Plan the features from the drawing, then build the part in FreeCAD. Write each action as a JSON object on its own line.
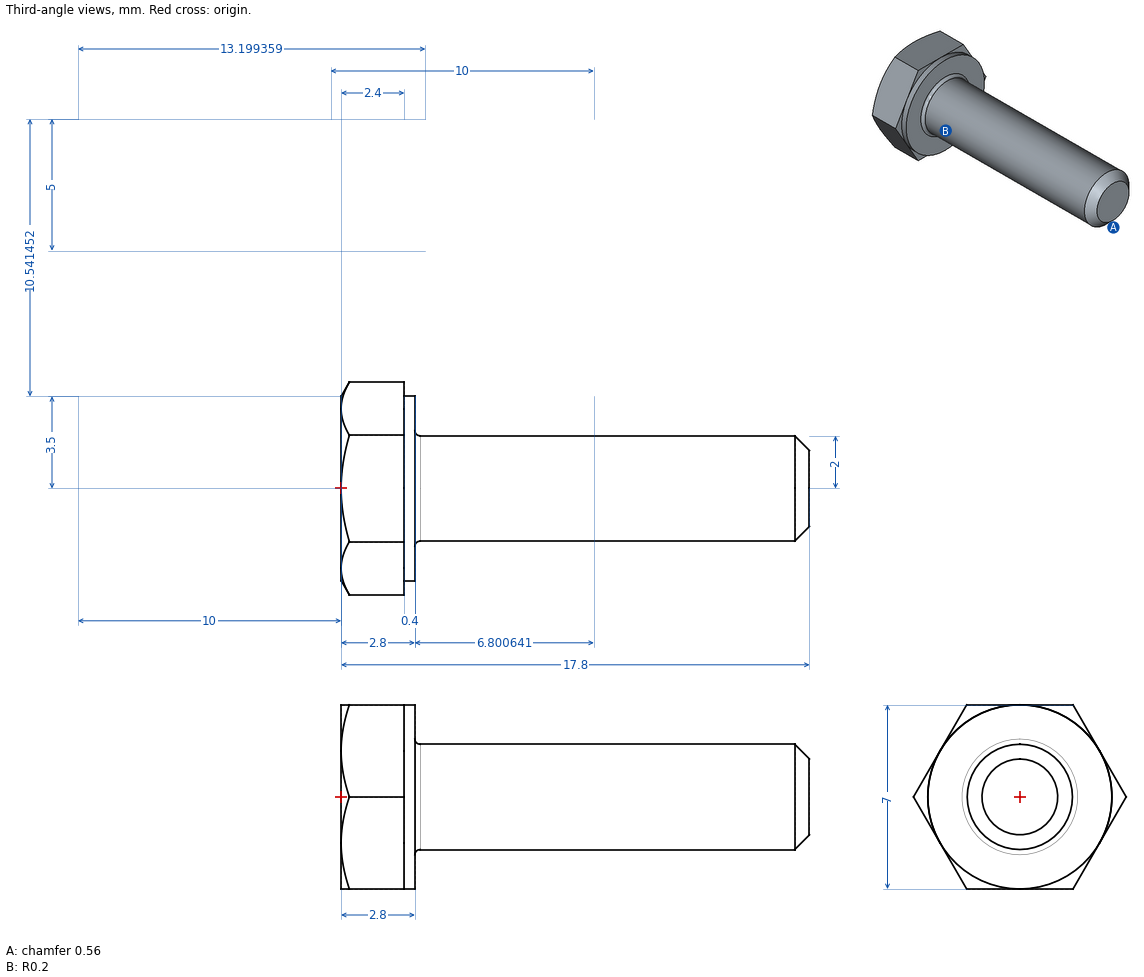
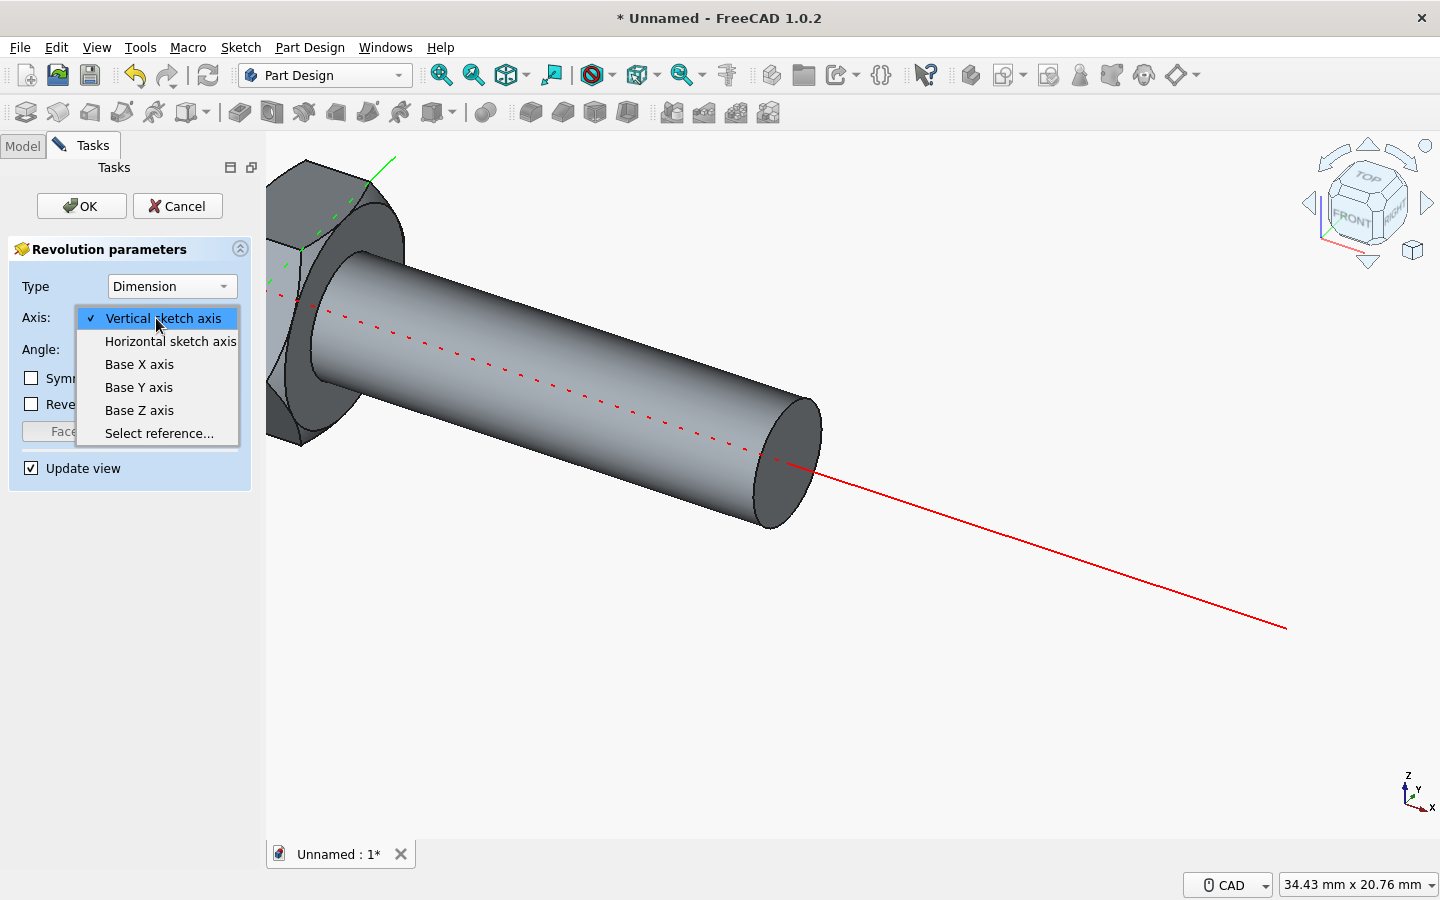
{"action": "left_click", "coordinate": [156, 342]}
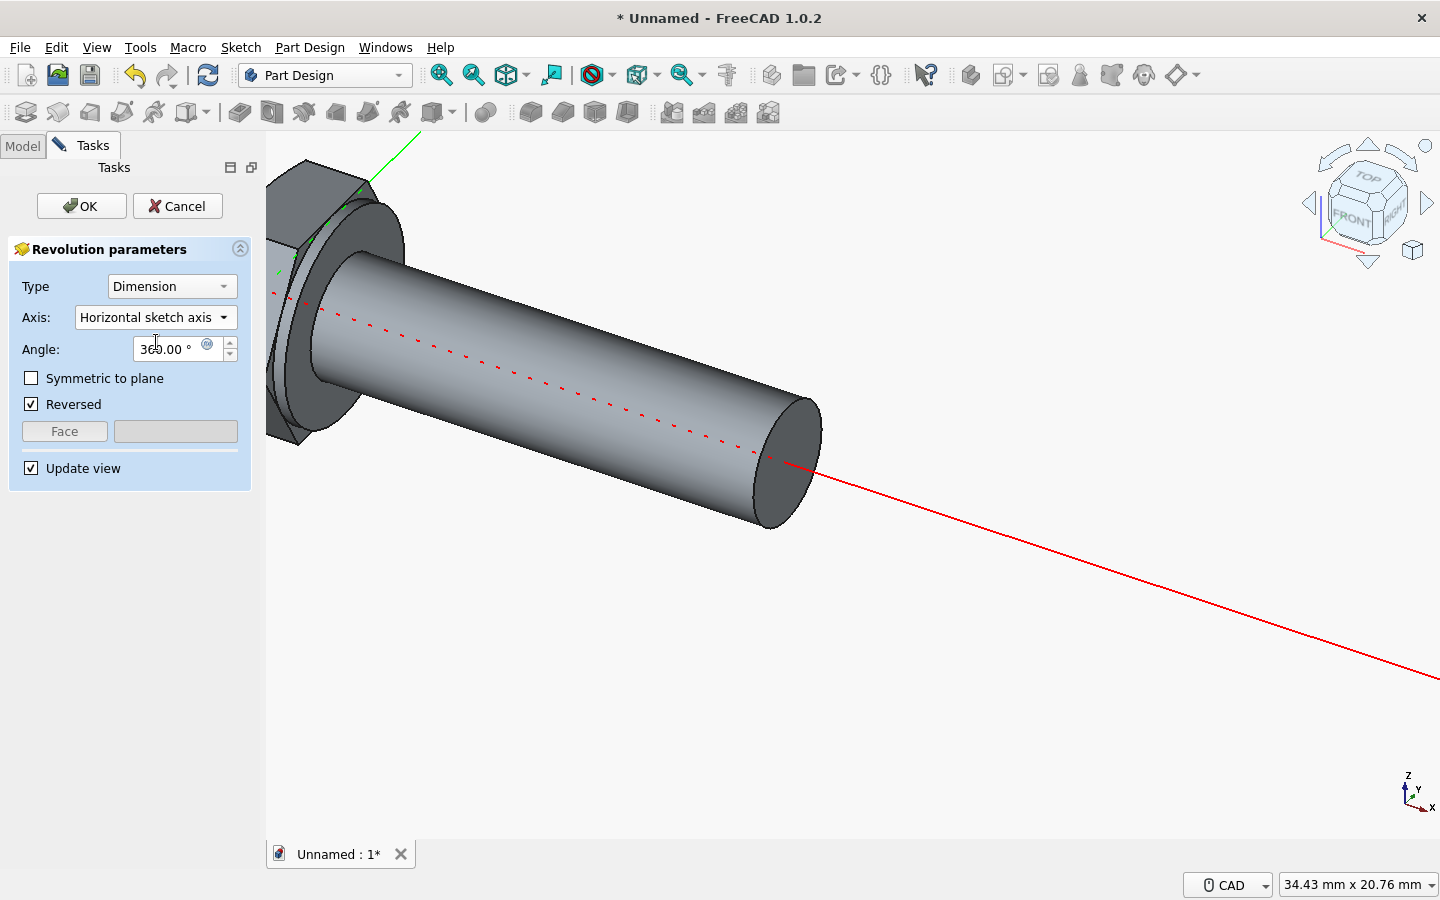
{"action": "left_click", "coordinate": [82, 206]}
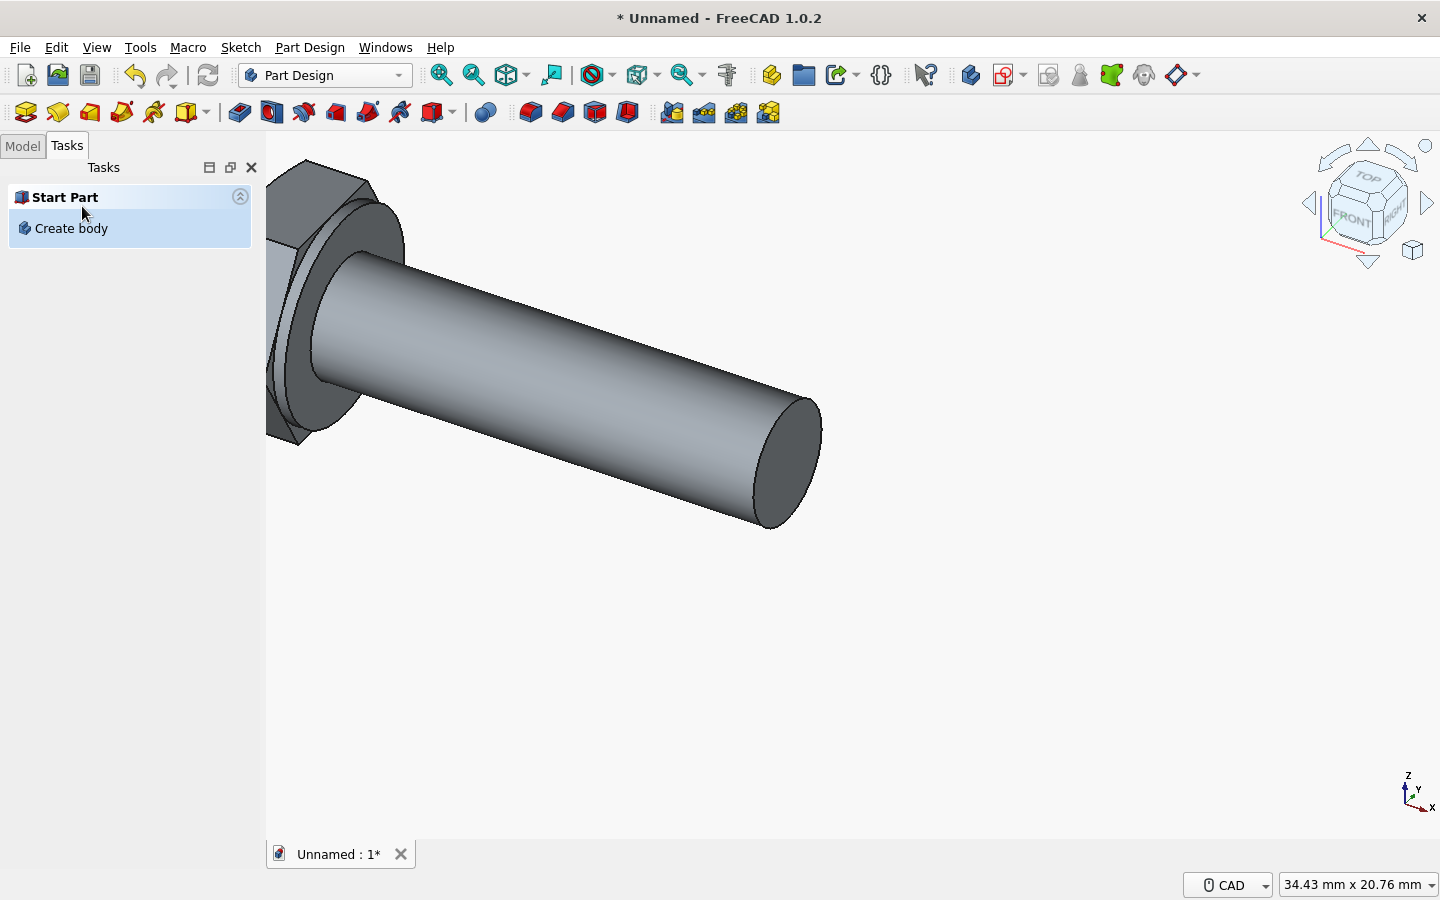
{"action": "left_click", "coordinate": [442, 76]}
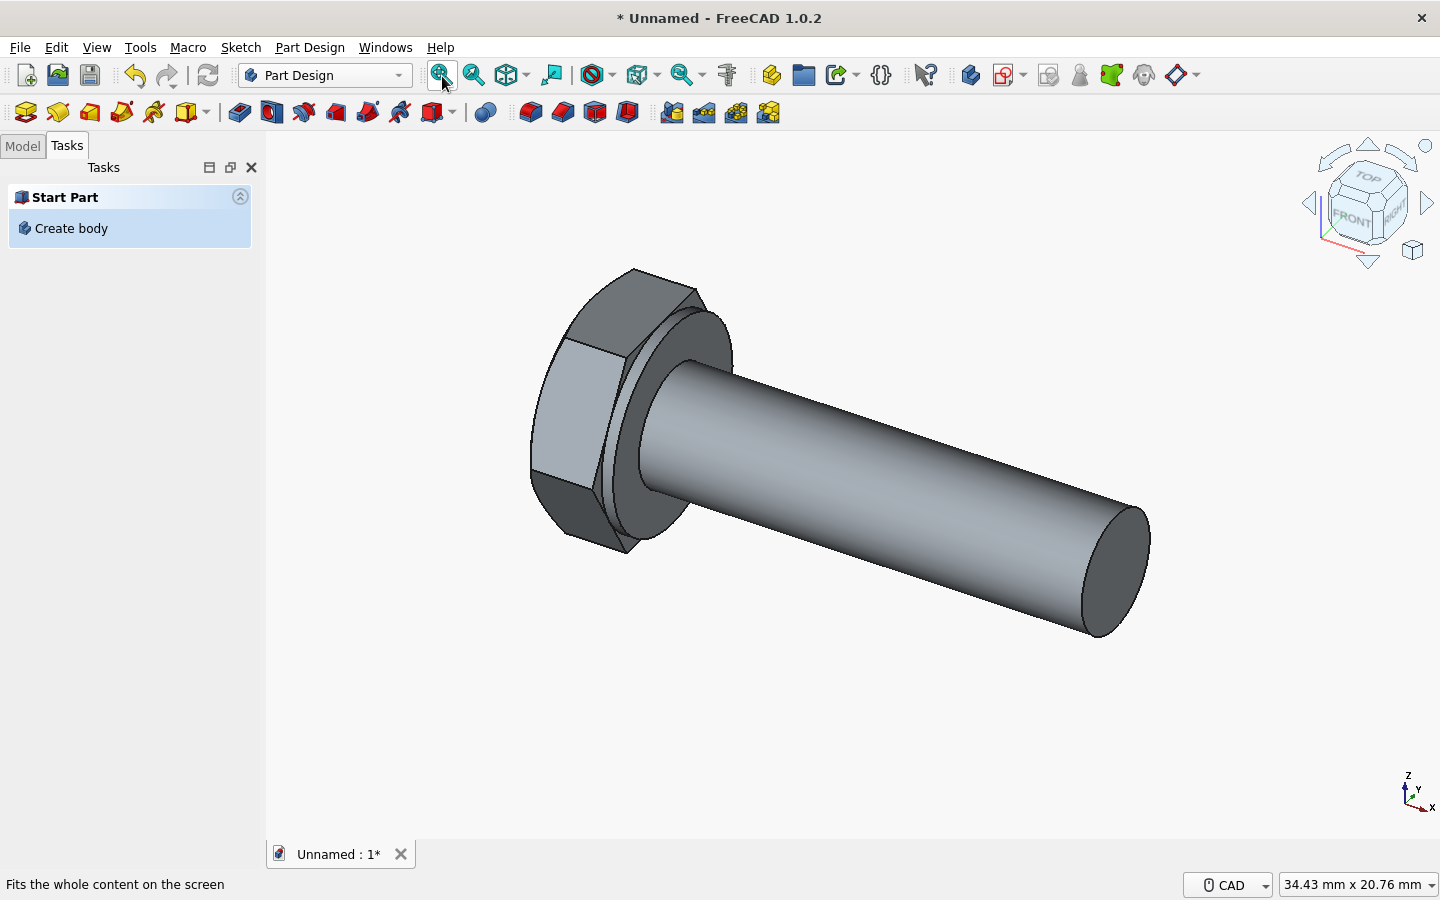
{"action": "left_click", "coordinate": [1082, 605]}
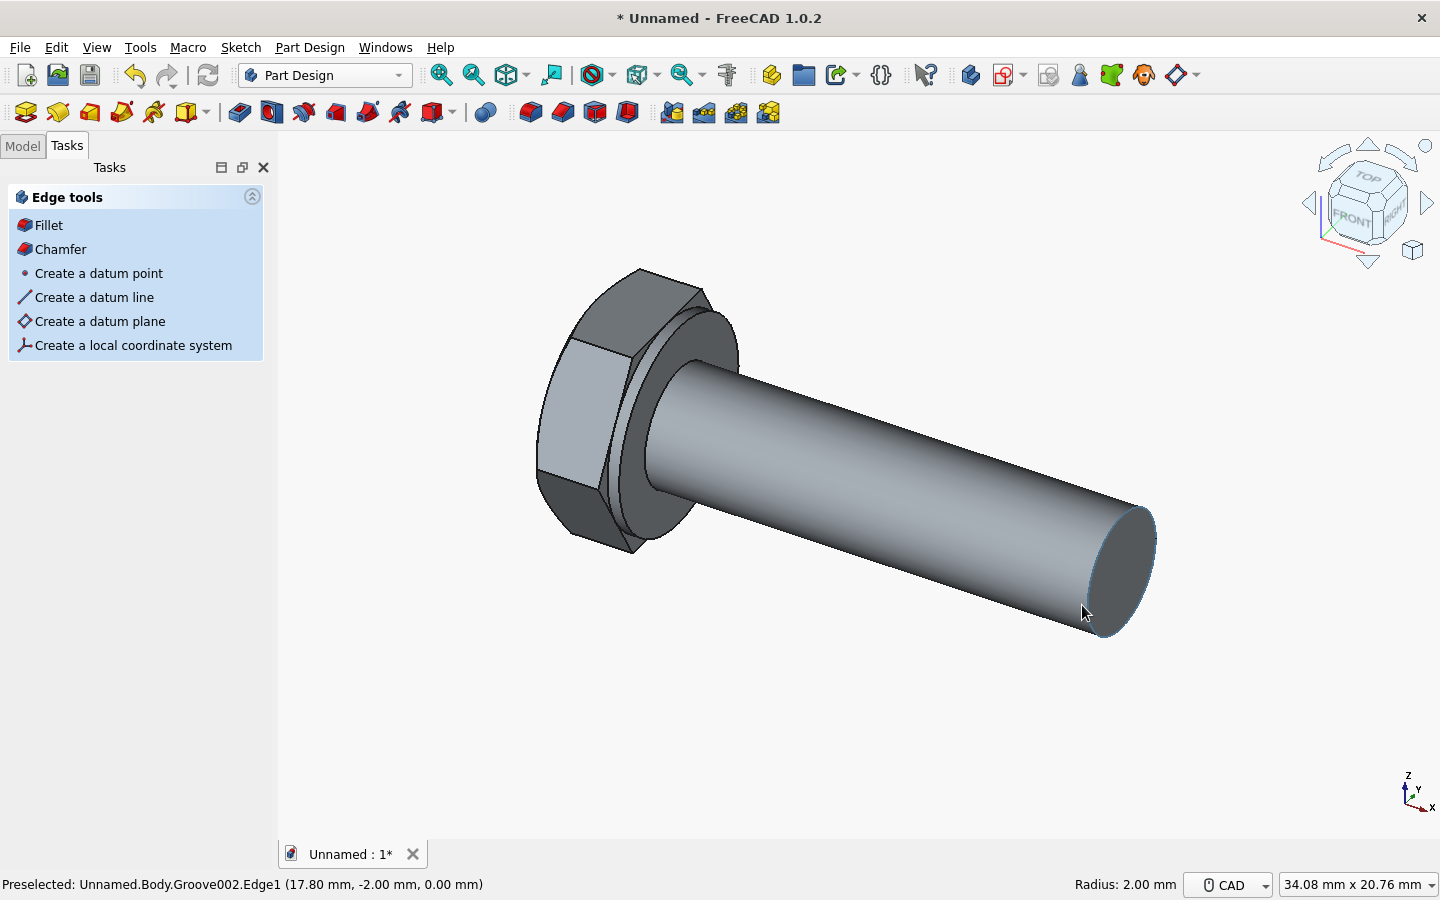
{"action": "left_click", "coordinate": [564, 112]}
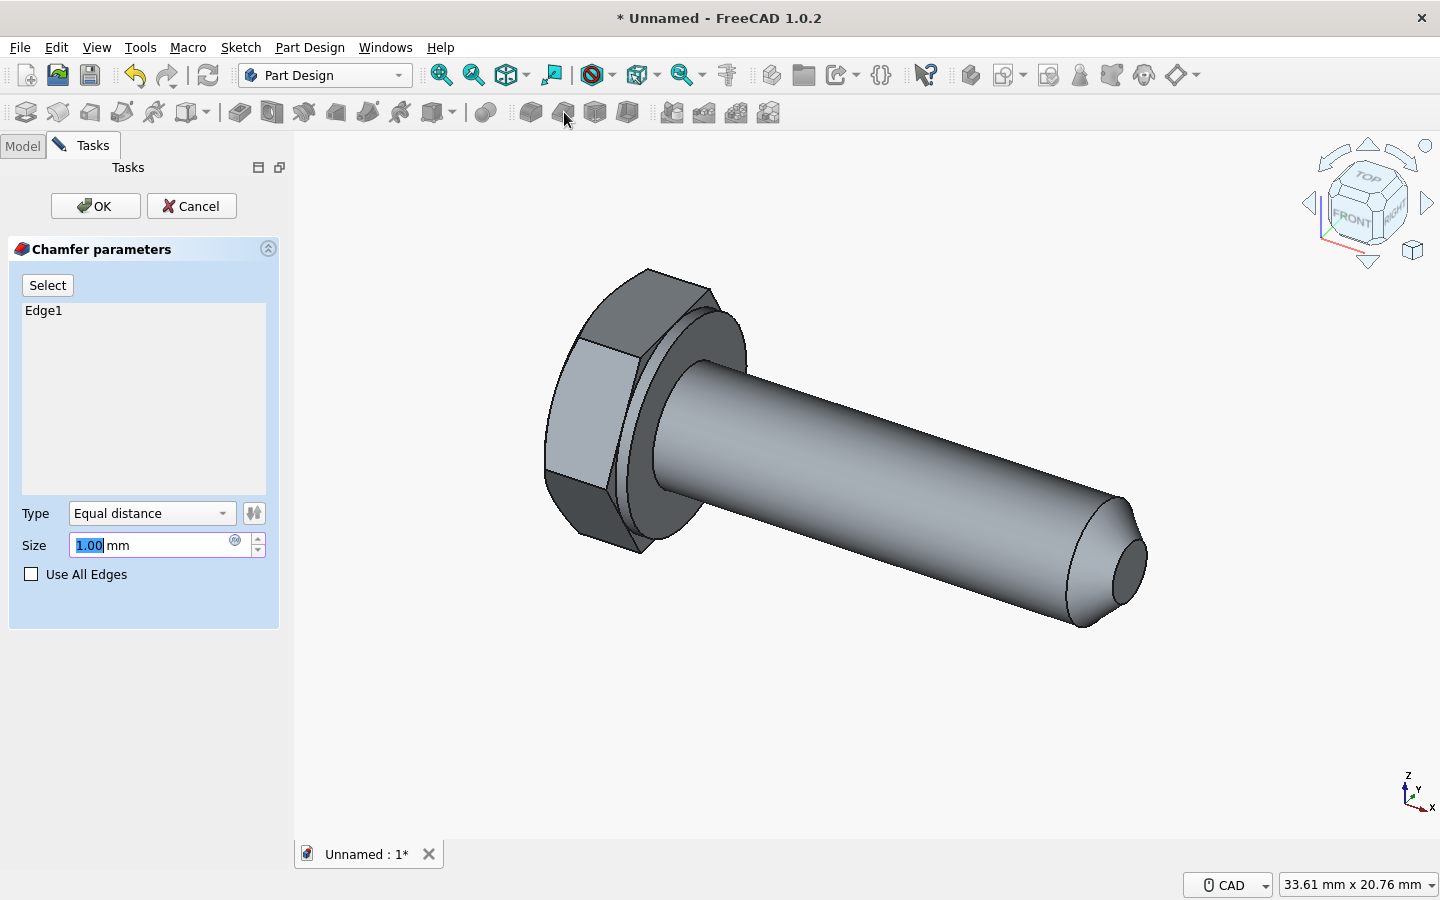
{"action": "type", "text": "0.56"}
{"action": "key", "text": "Tab"}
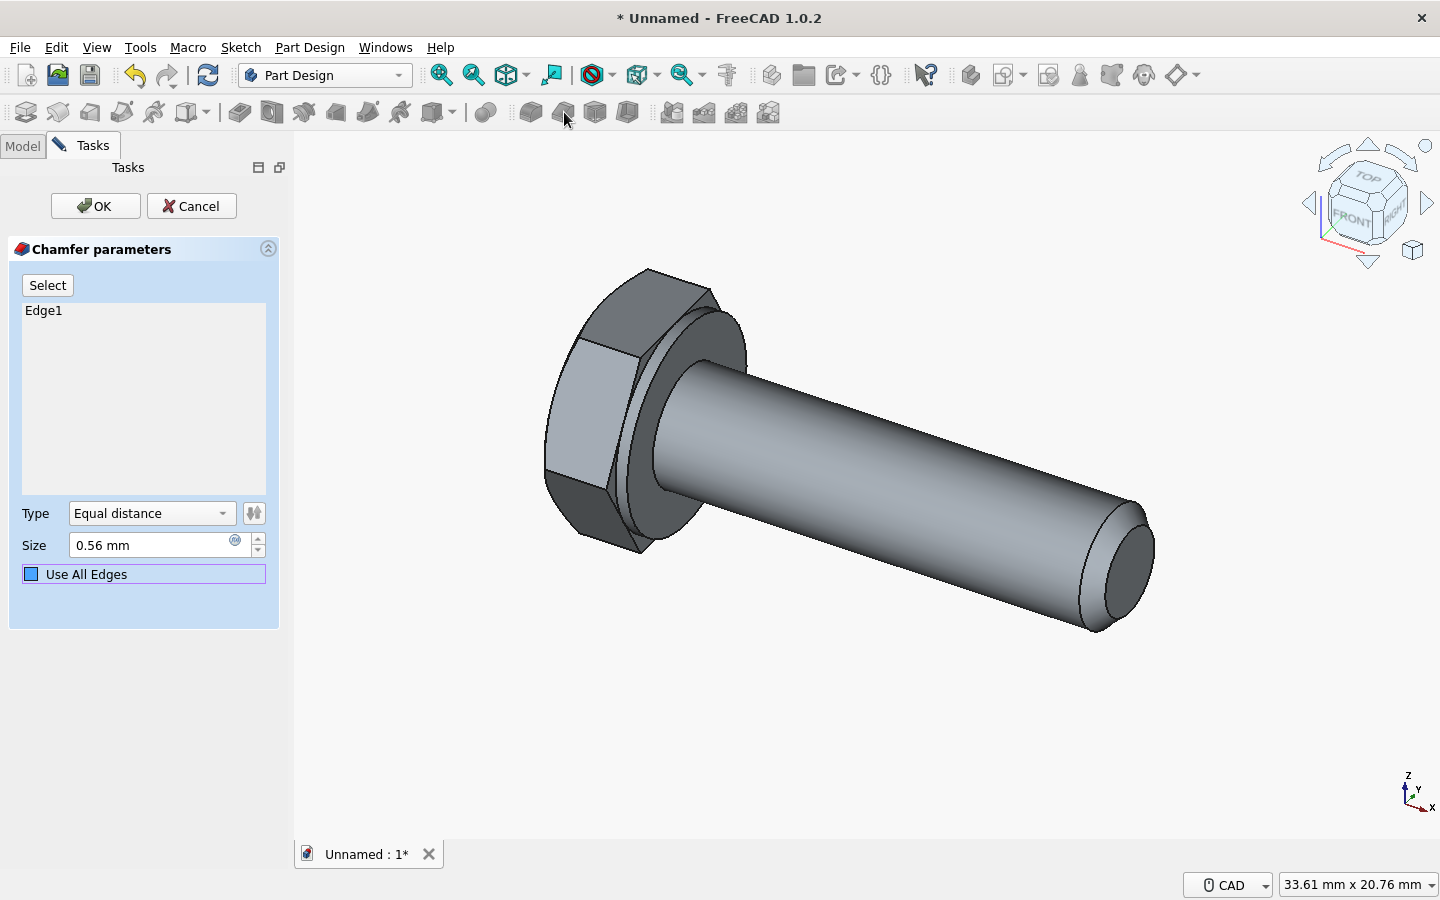
{"action": "left_click", "coordinate": [96, 206]}